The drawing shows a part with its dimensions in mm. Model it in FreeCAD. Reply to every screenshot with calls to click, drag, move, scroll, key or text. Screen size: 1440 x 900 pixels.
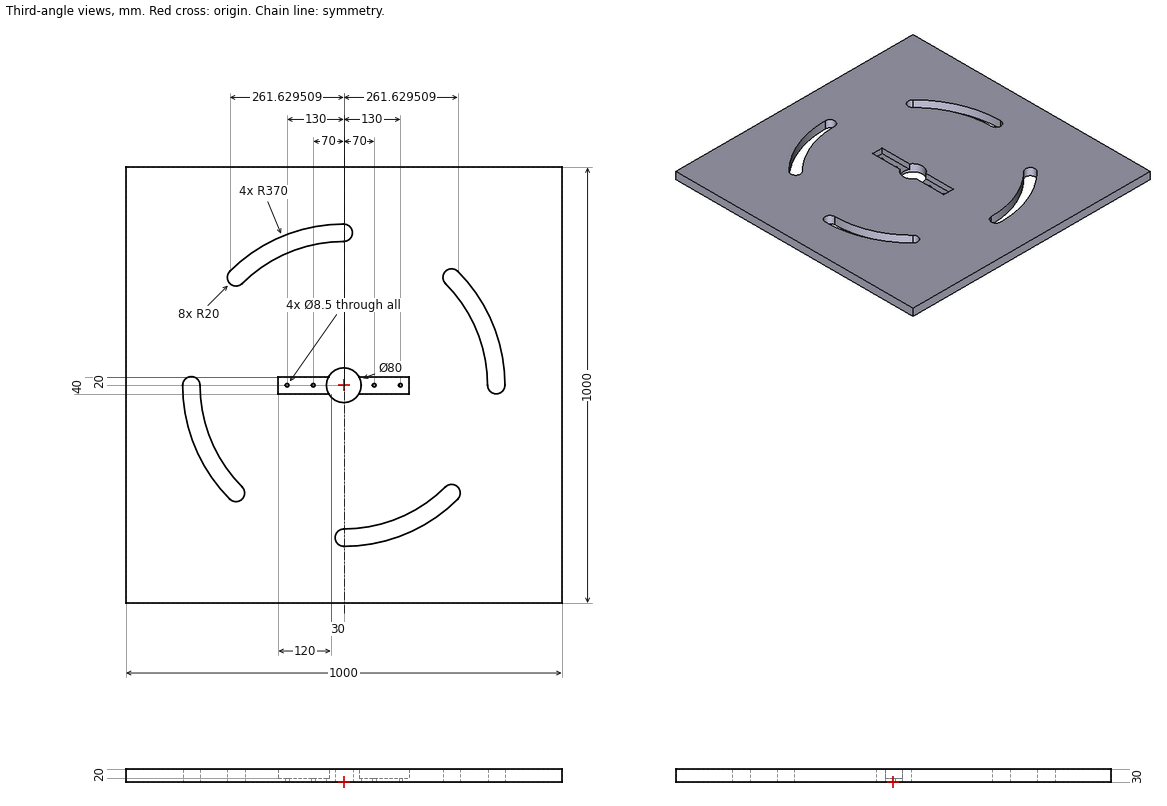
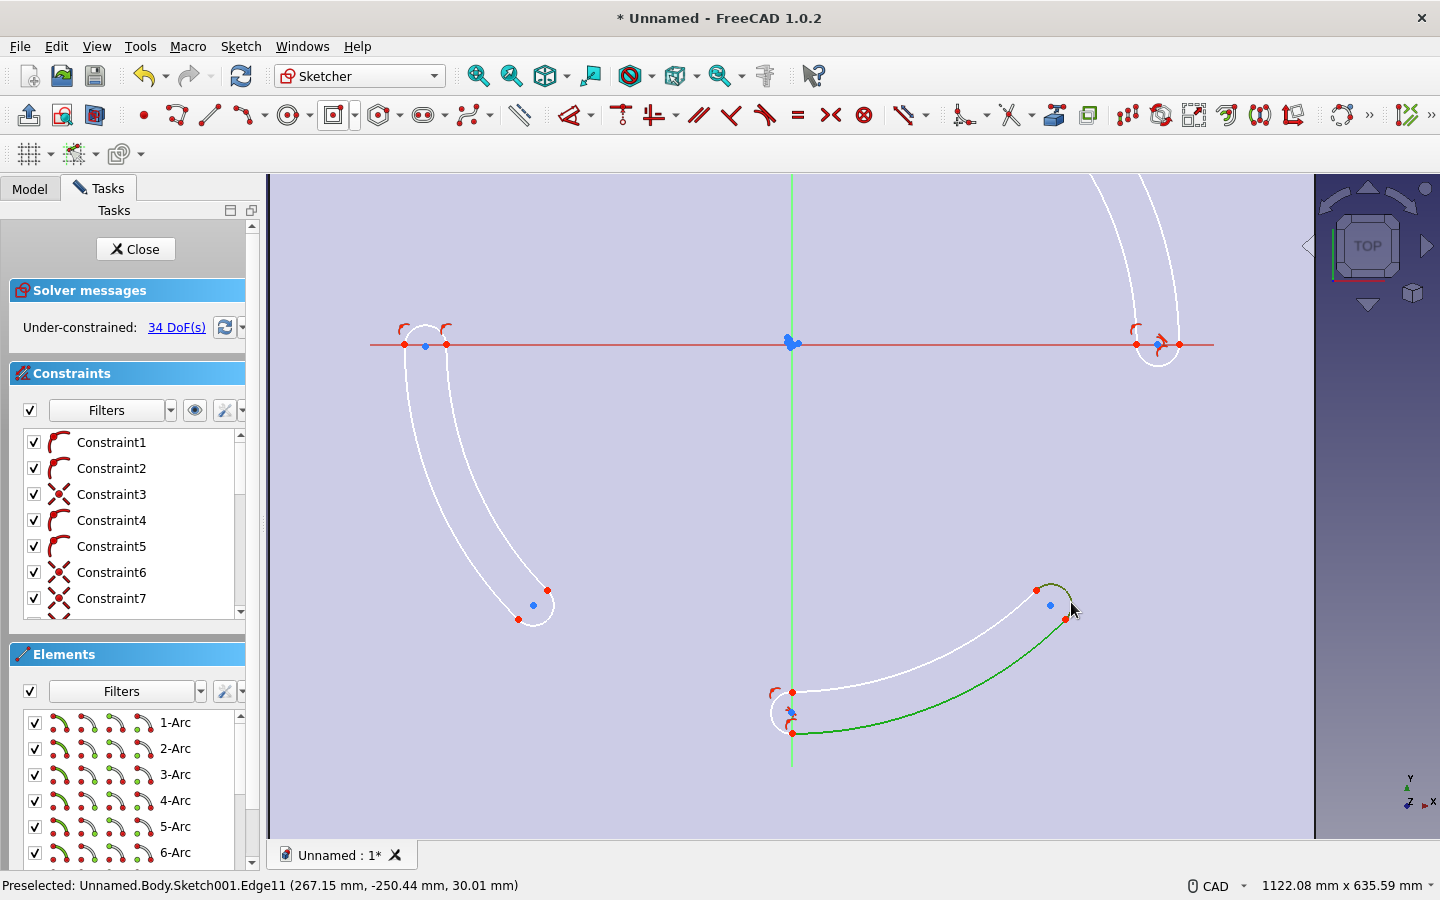
key(t)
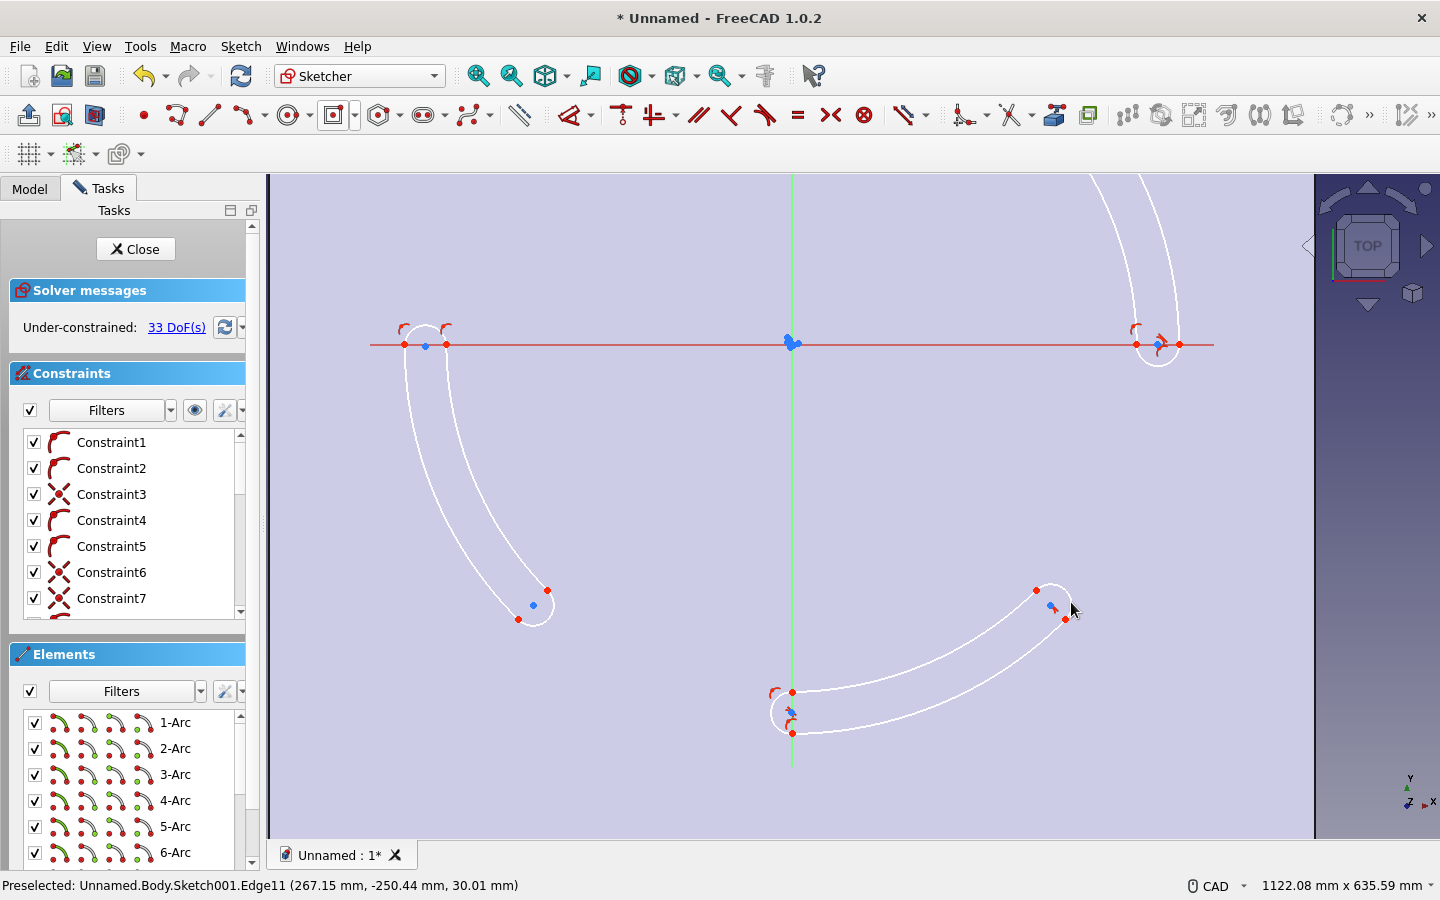
click(1071, 602)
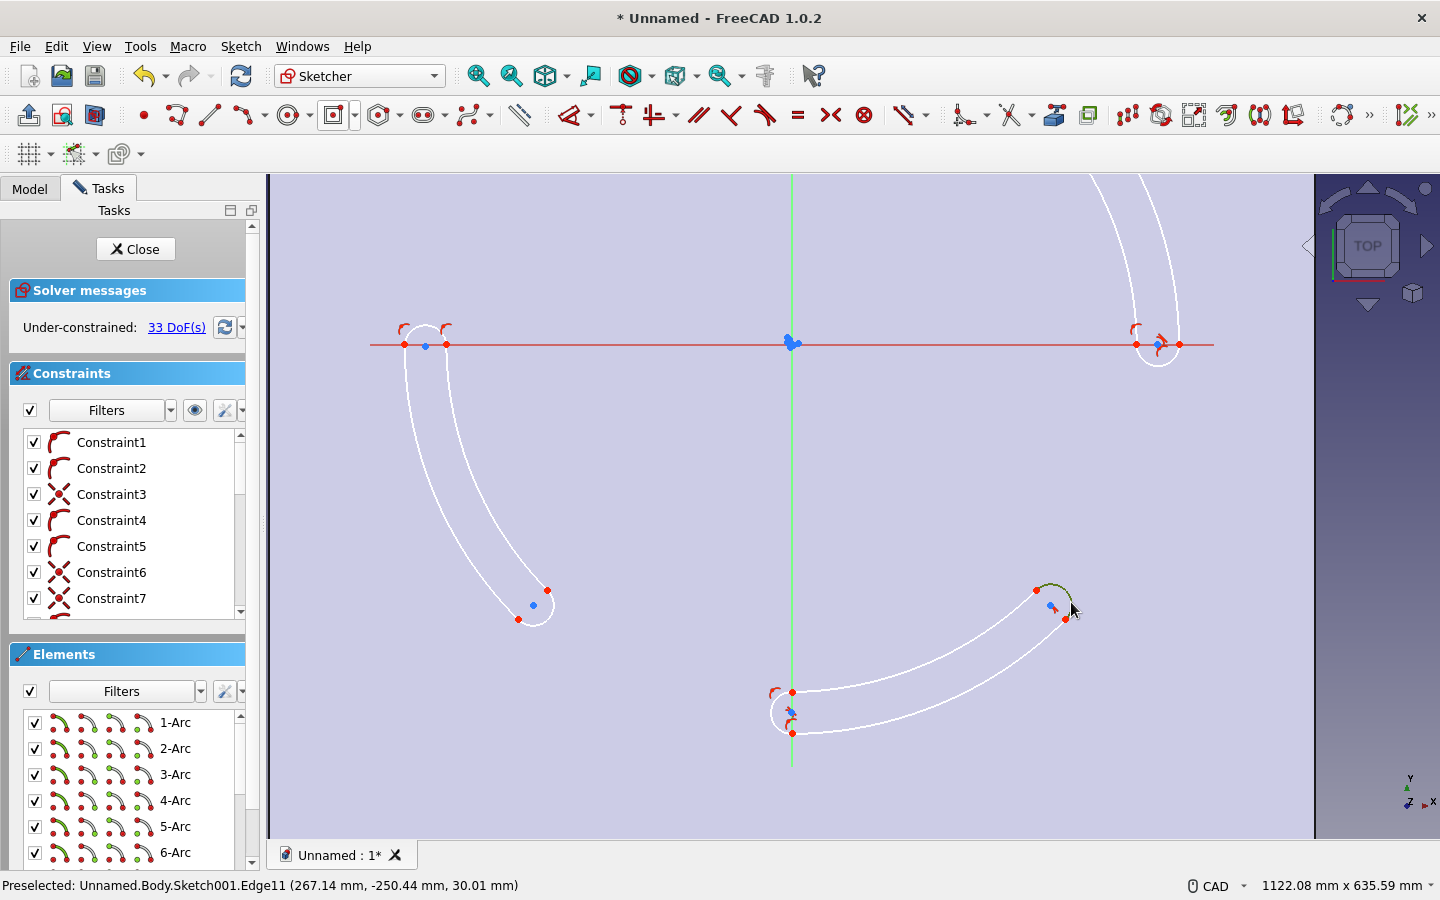
click(873, 682)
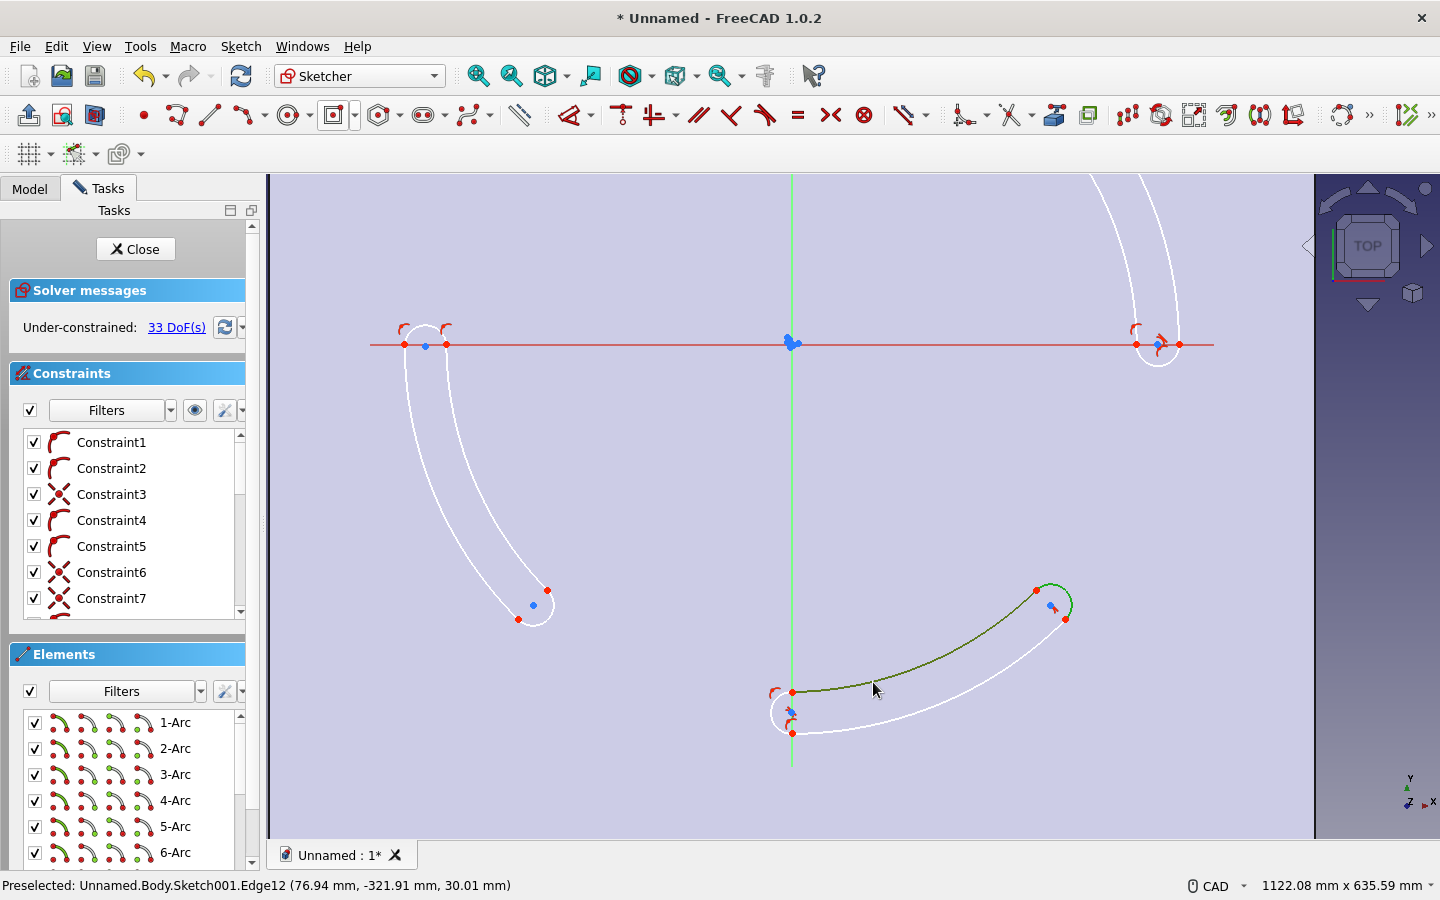
key(t)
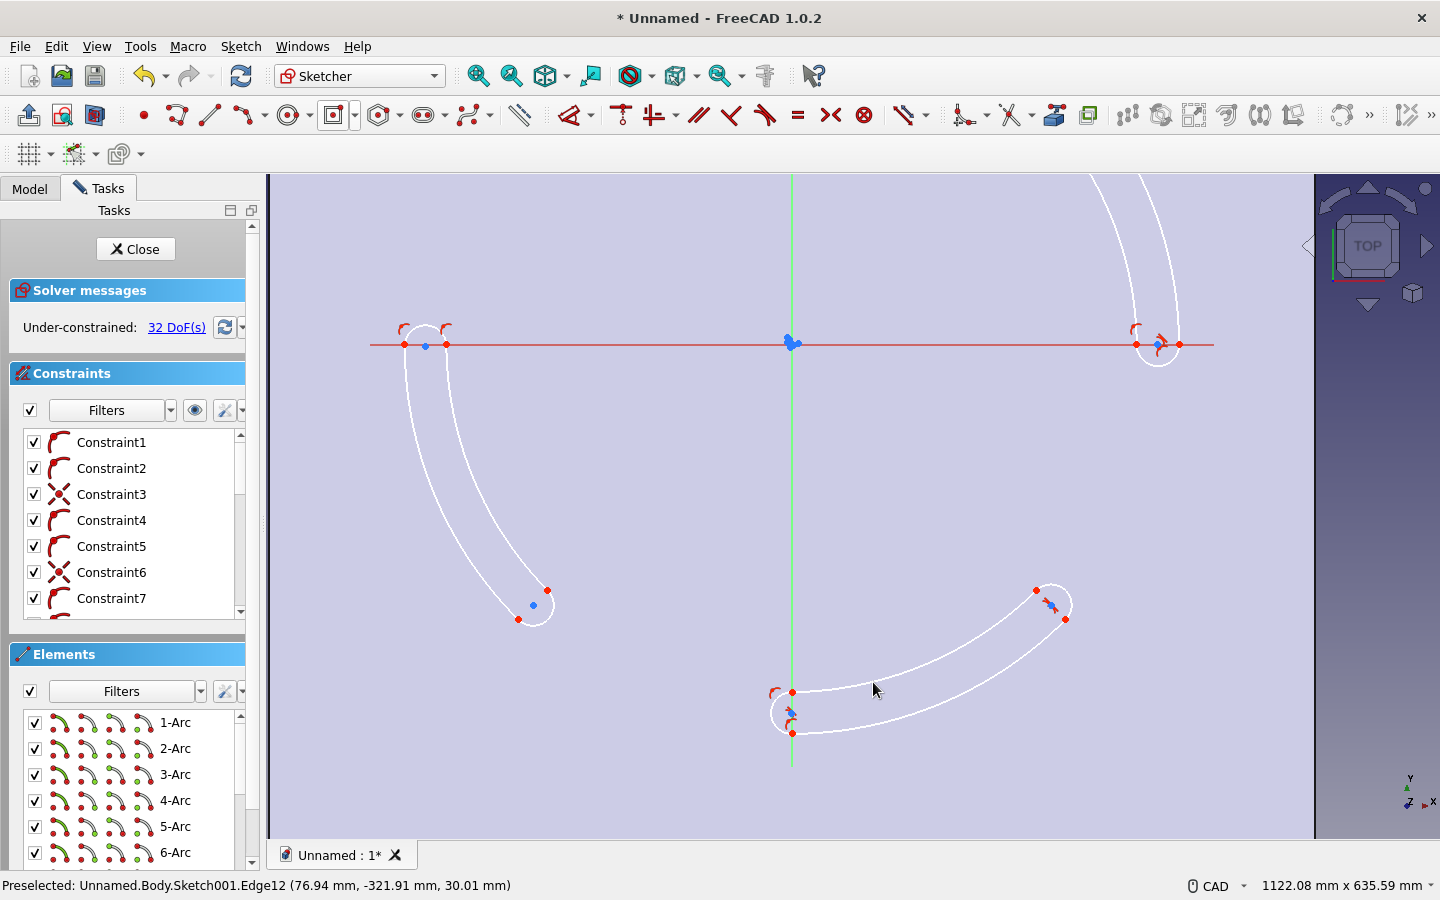
click(437, 329)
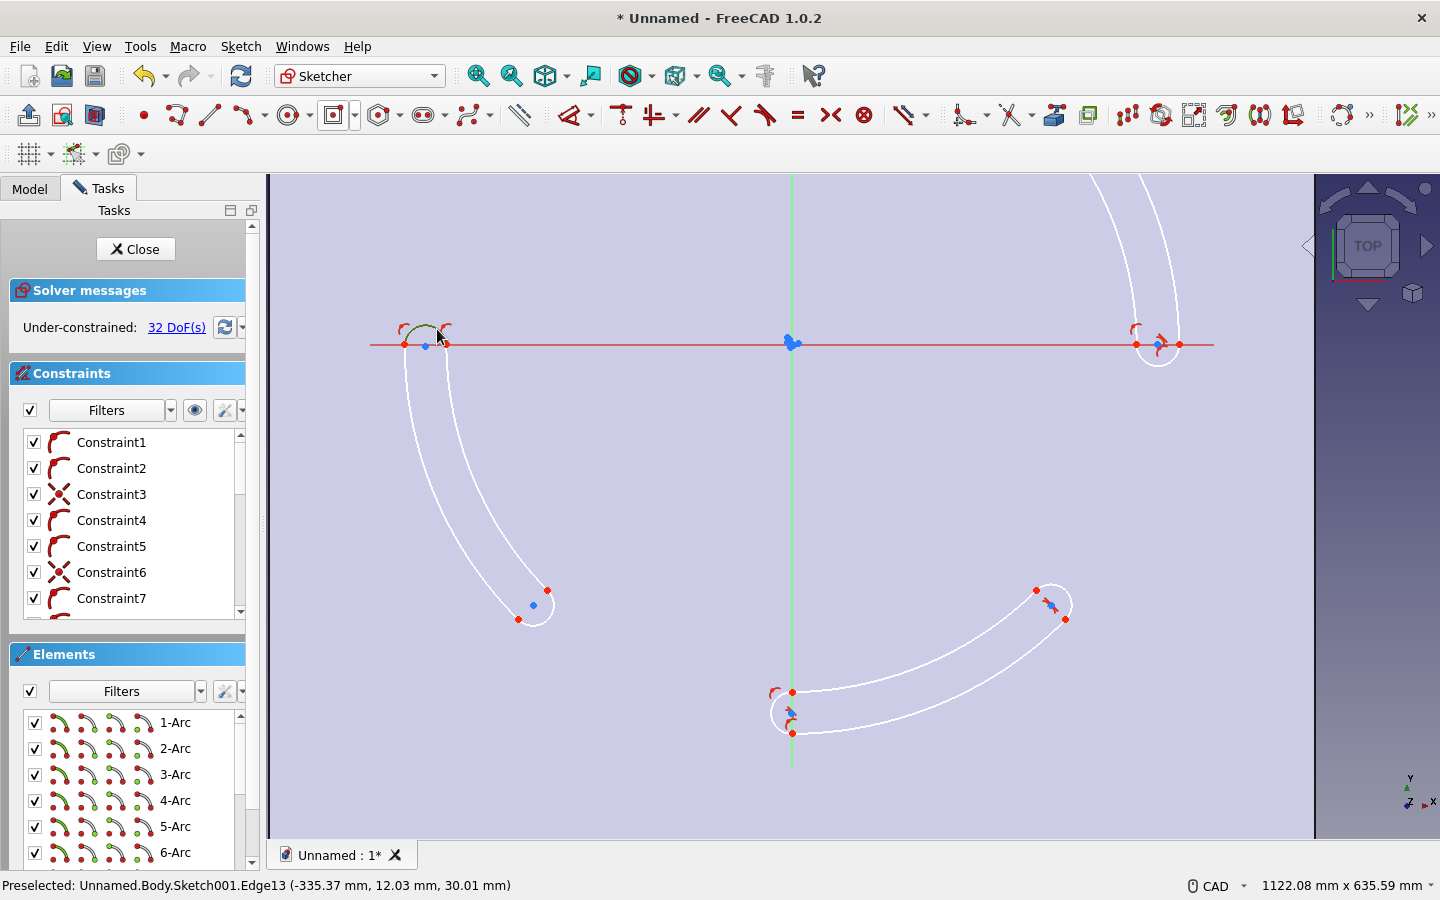
click(415, 436)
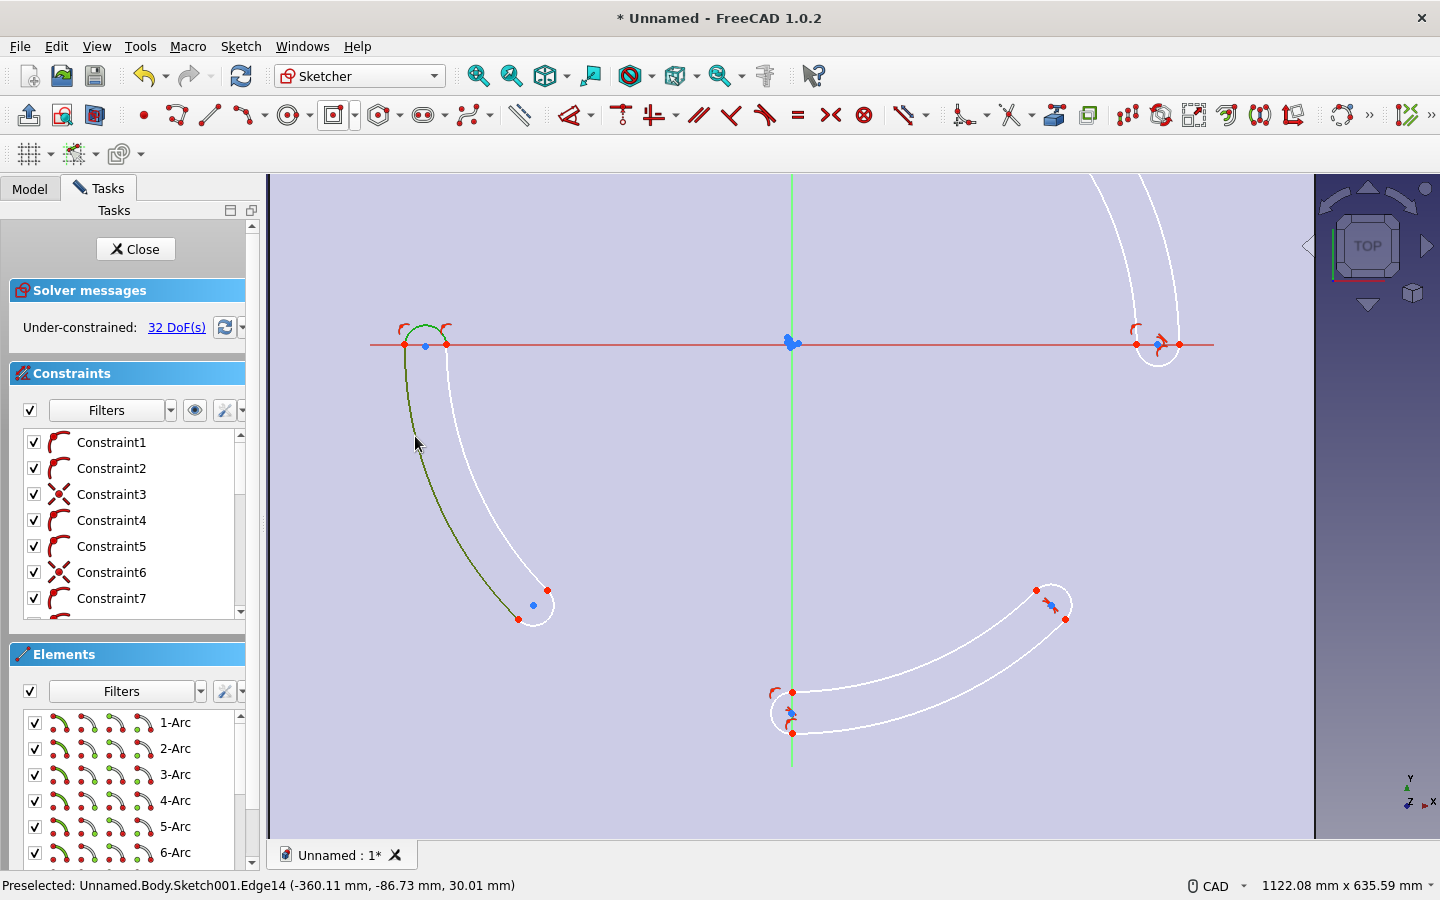
click(765, 116)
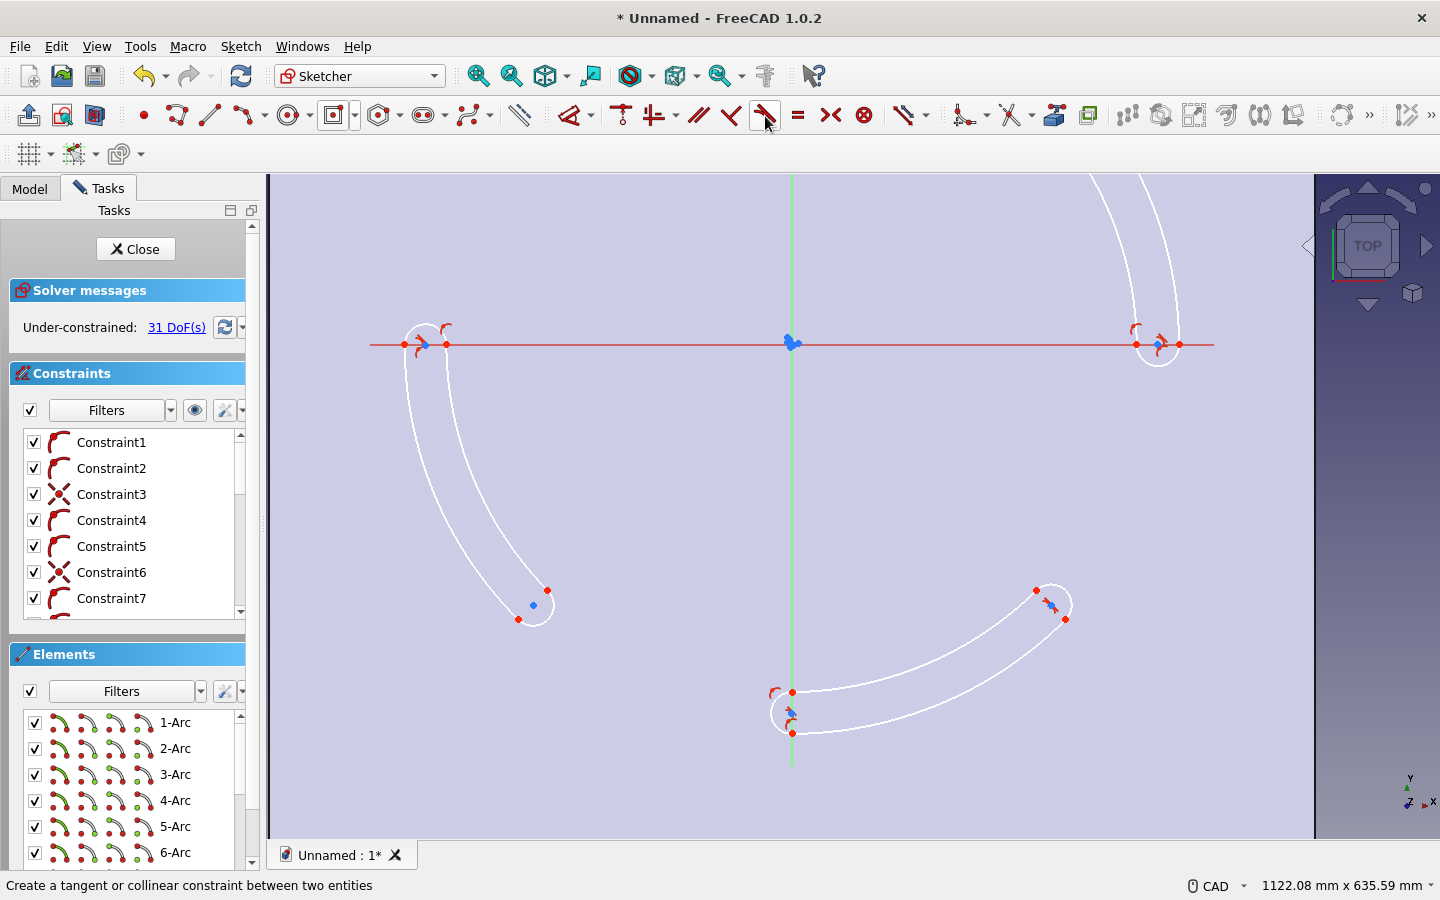
click(415, 436)